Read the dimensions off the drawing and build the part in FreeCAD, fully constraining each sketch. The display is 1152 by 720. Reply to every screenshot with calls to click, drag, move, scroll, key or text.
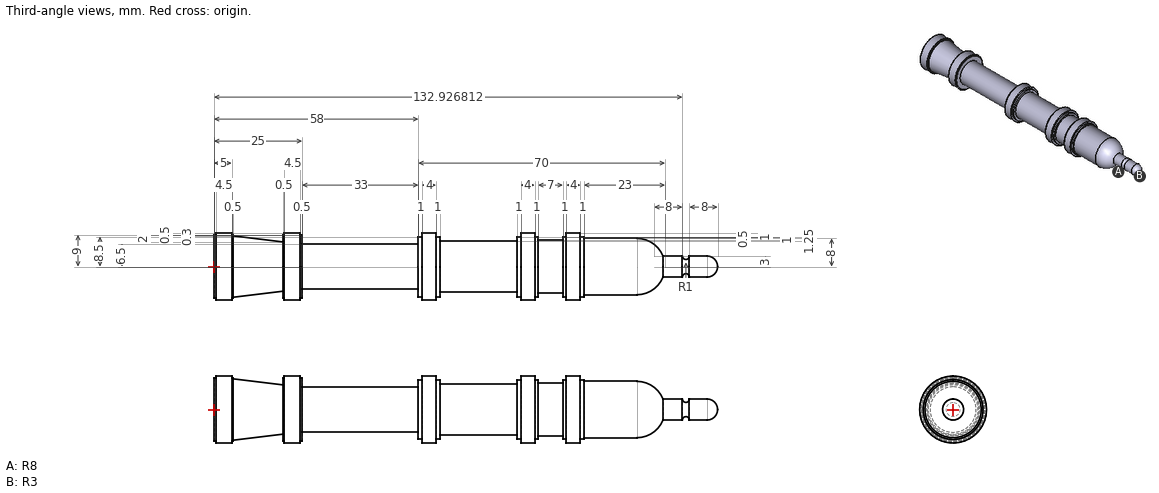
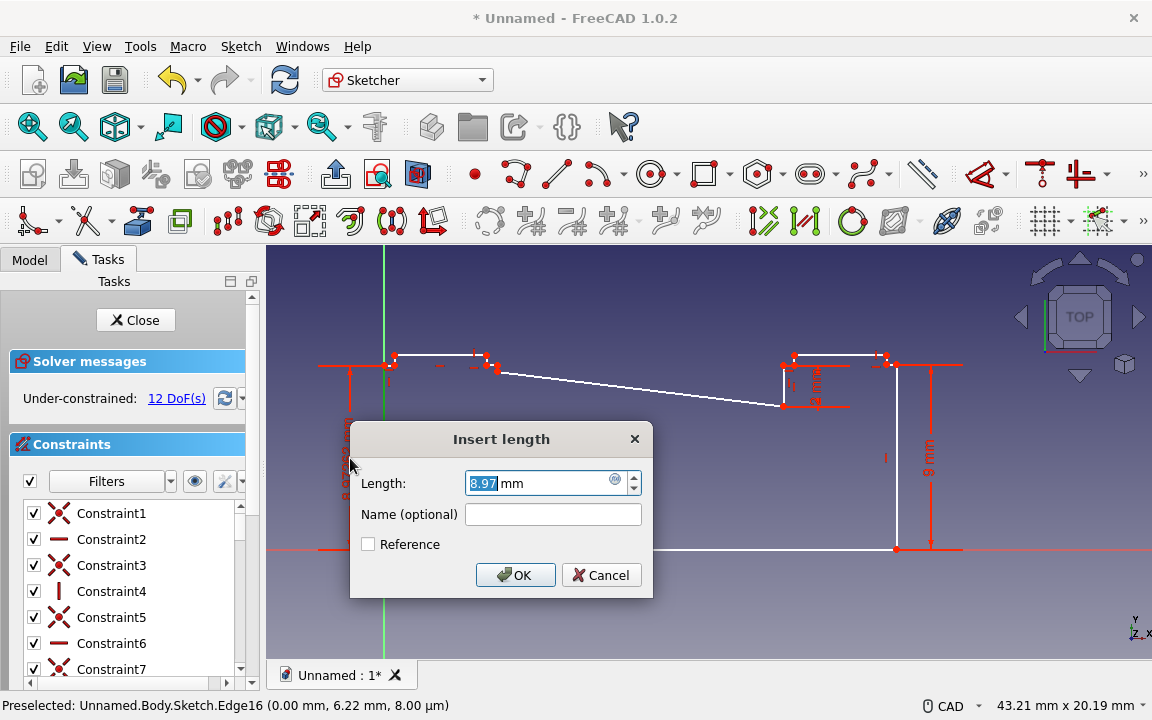
text(9)
key(Return)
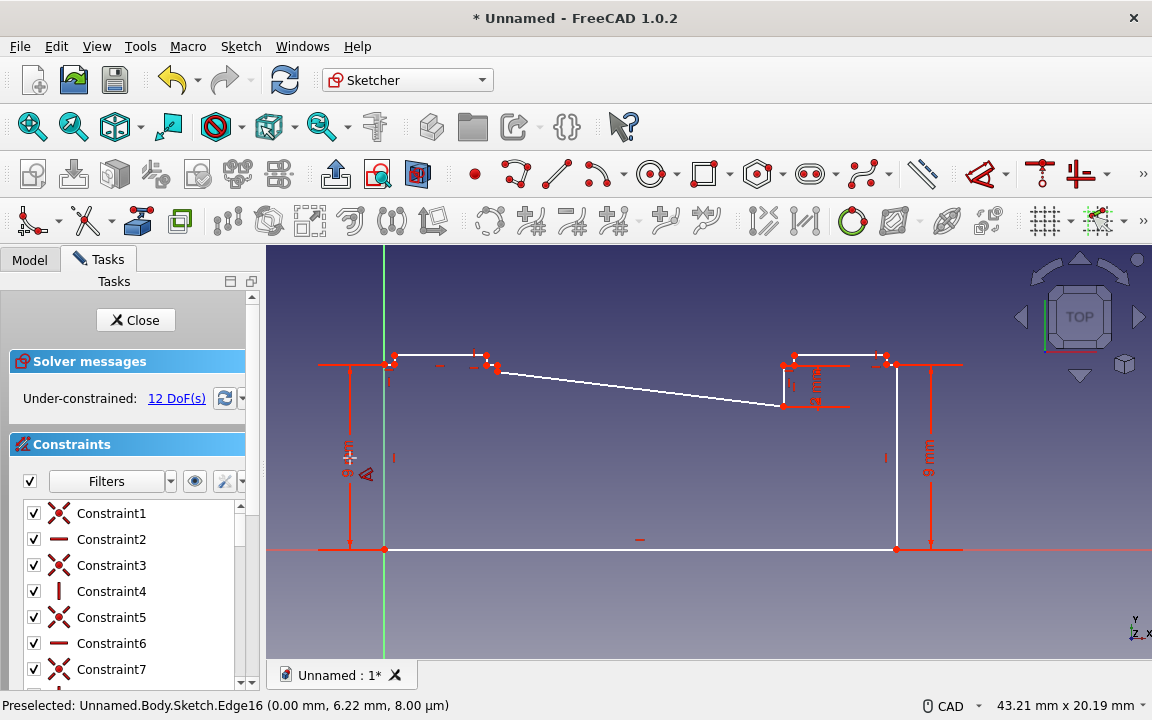
click(538, 550)
click(641, 584)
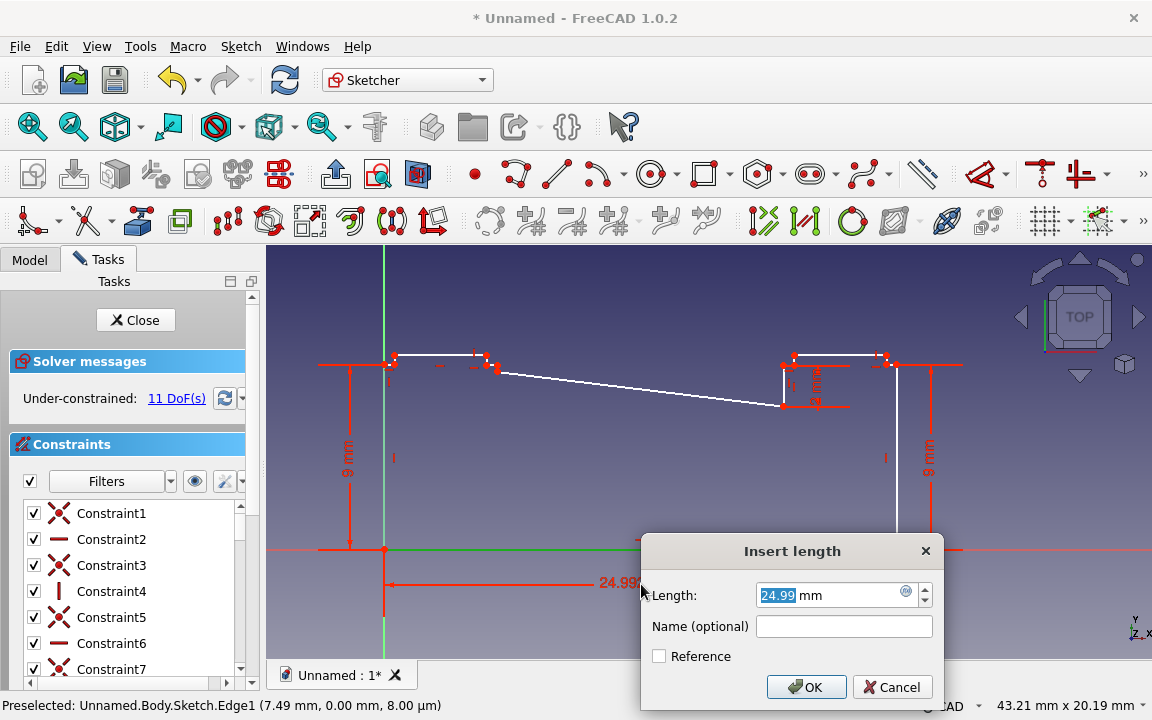
text(25)
key(Return)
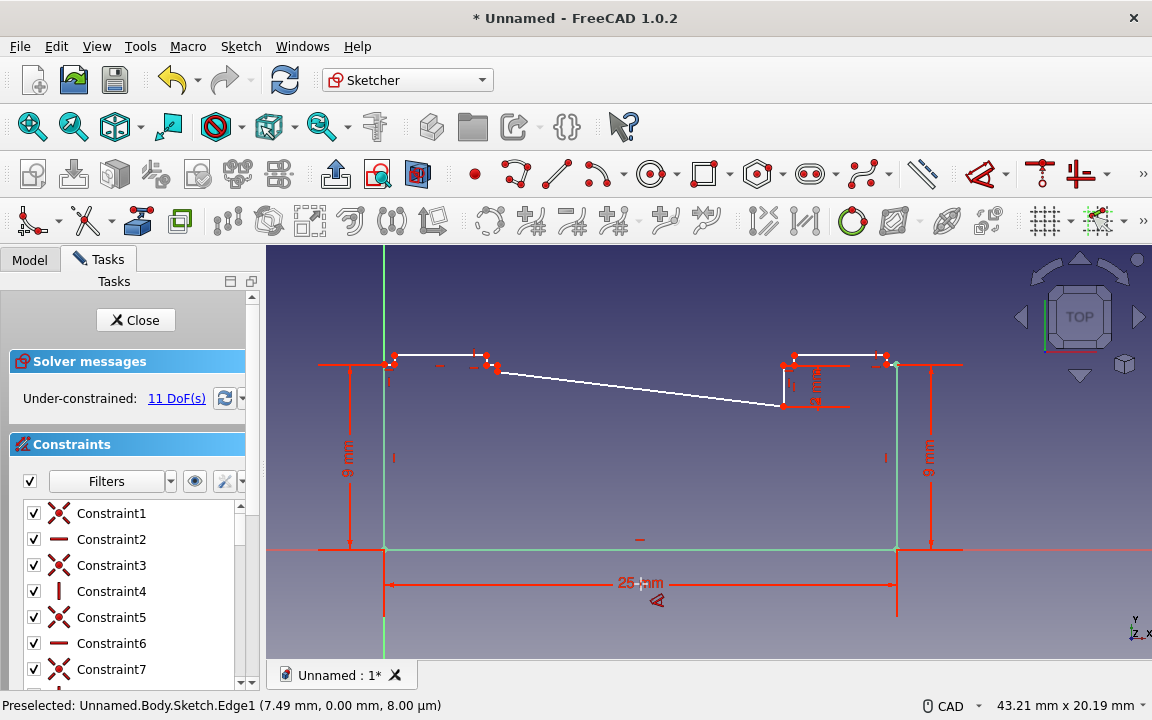
click(794, 366)
click(350, 415)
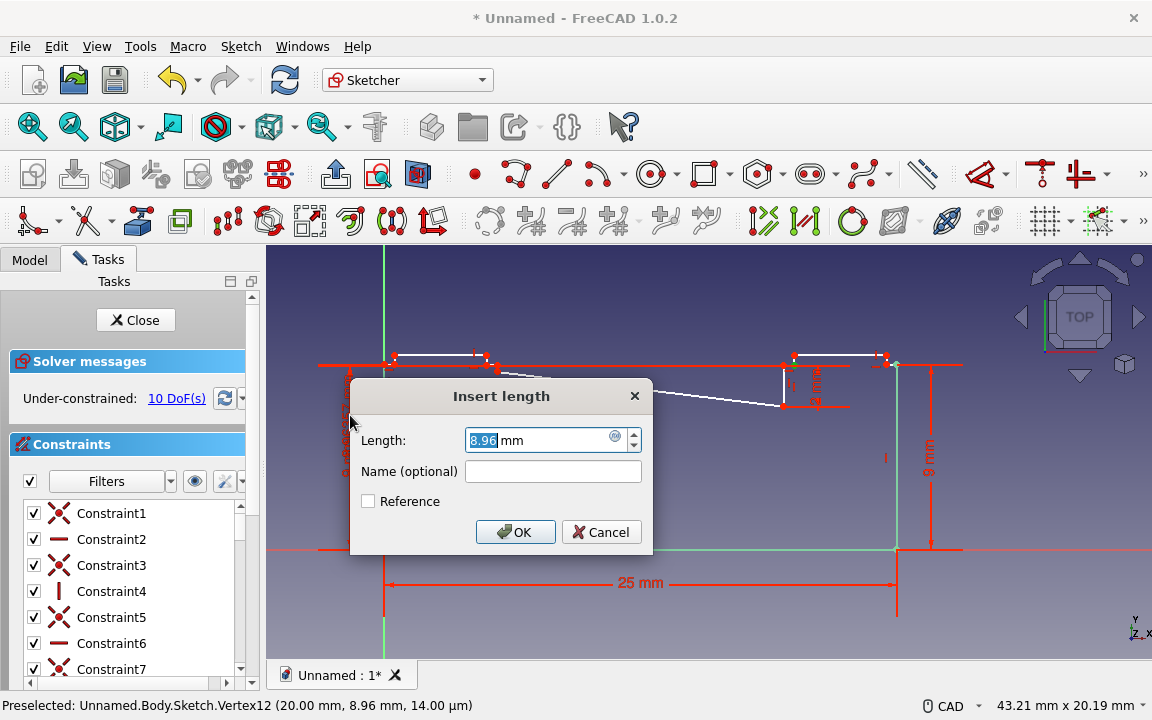
text(9)
key(Return)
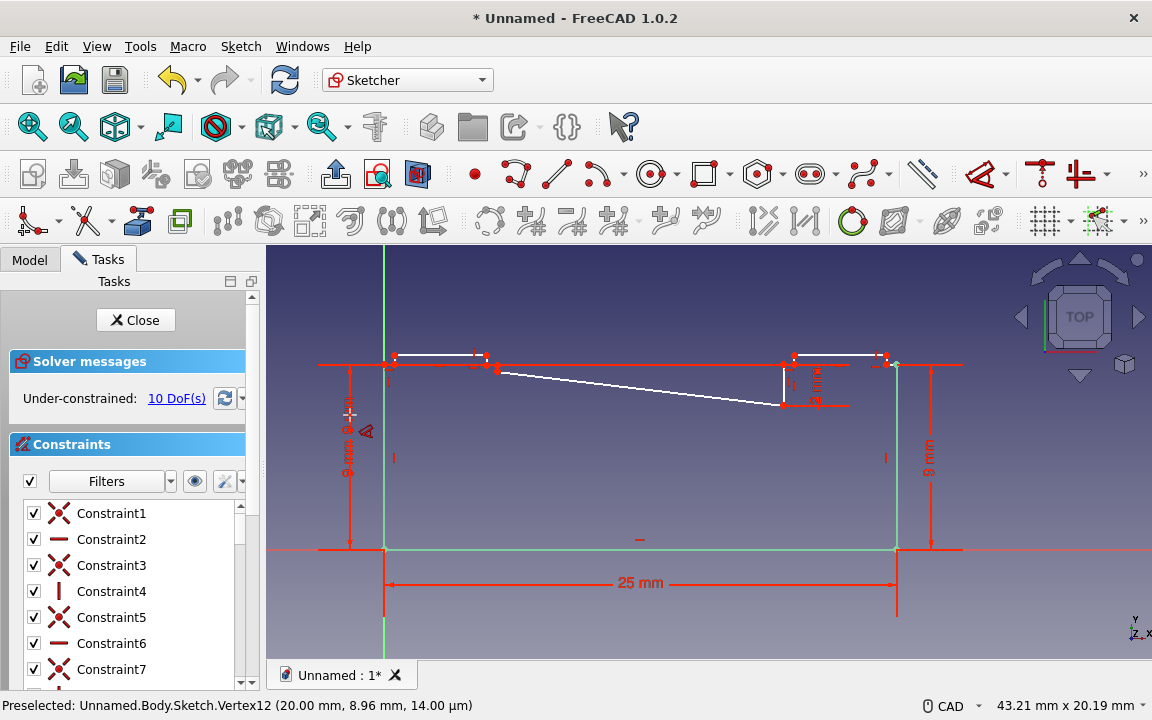
scroll(497, 365, up, 3)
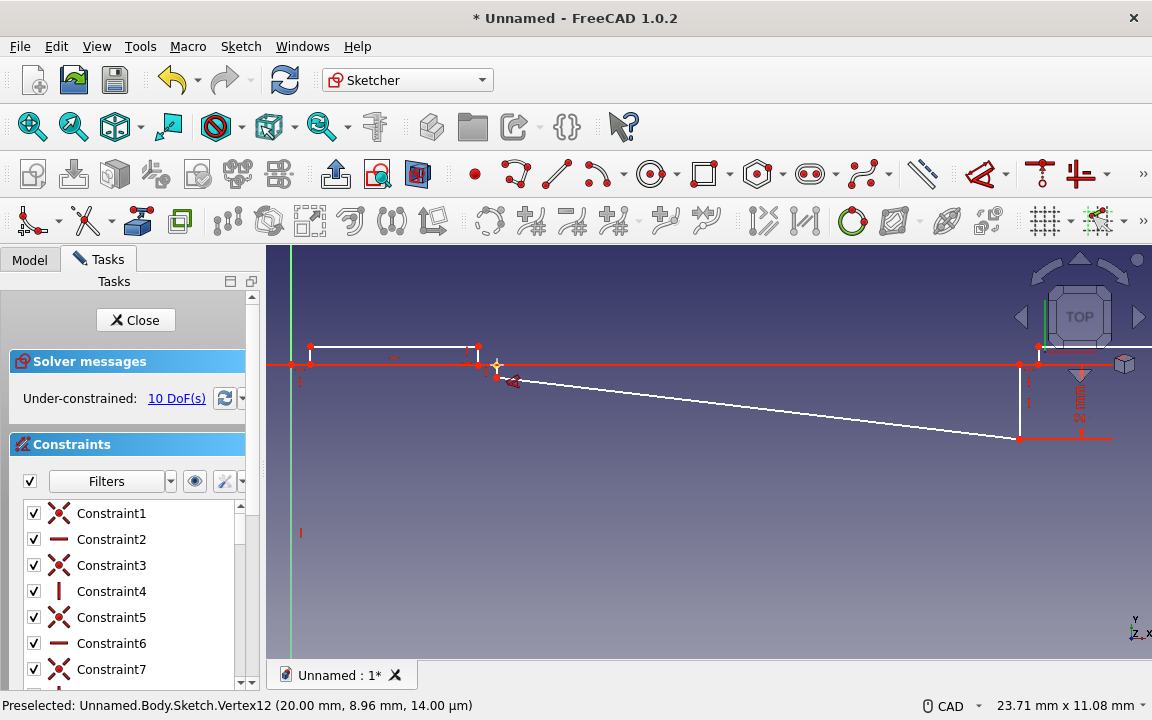
click(497, 365)
click(531, 498)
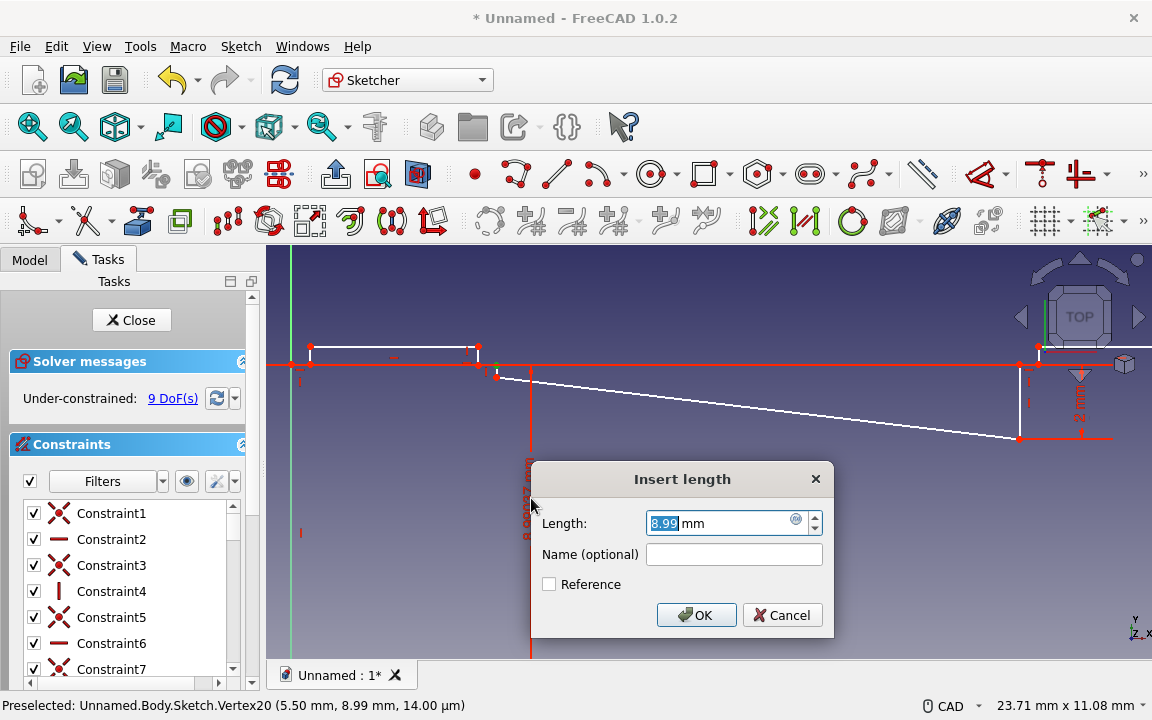
text(9)
key(Return)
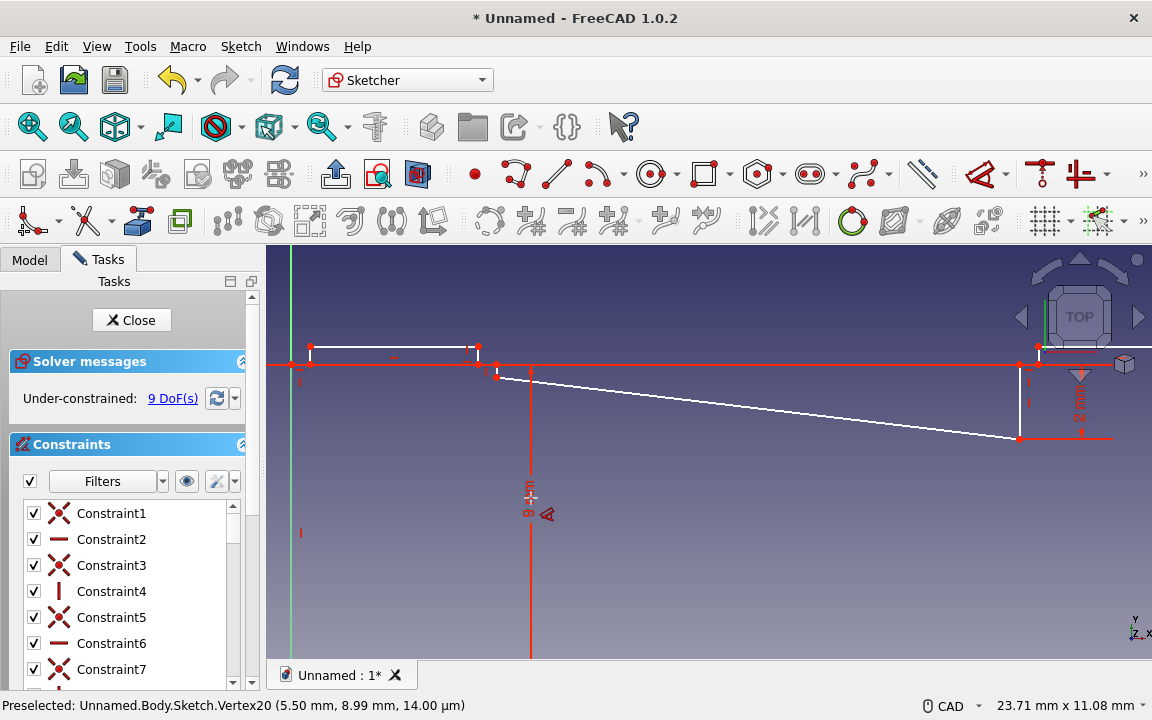
click(478, 365)
click(386, 331)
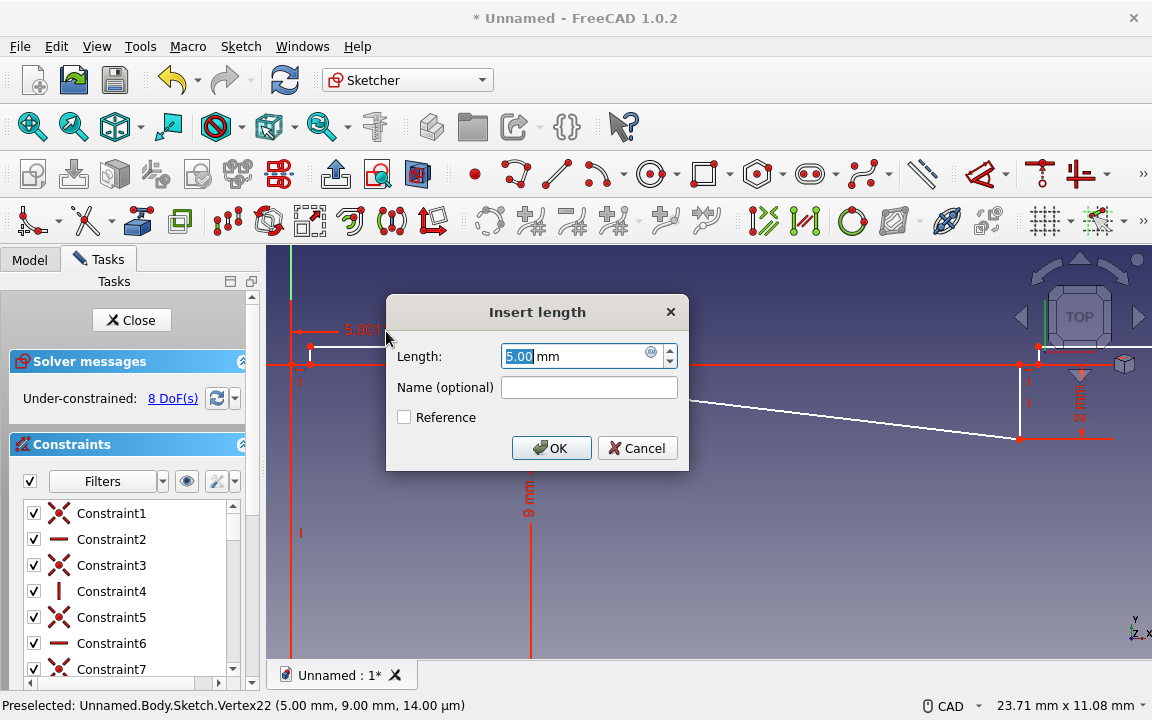
text(5)
key(Return)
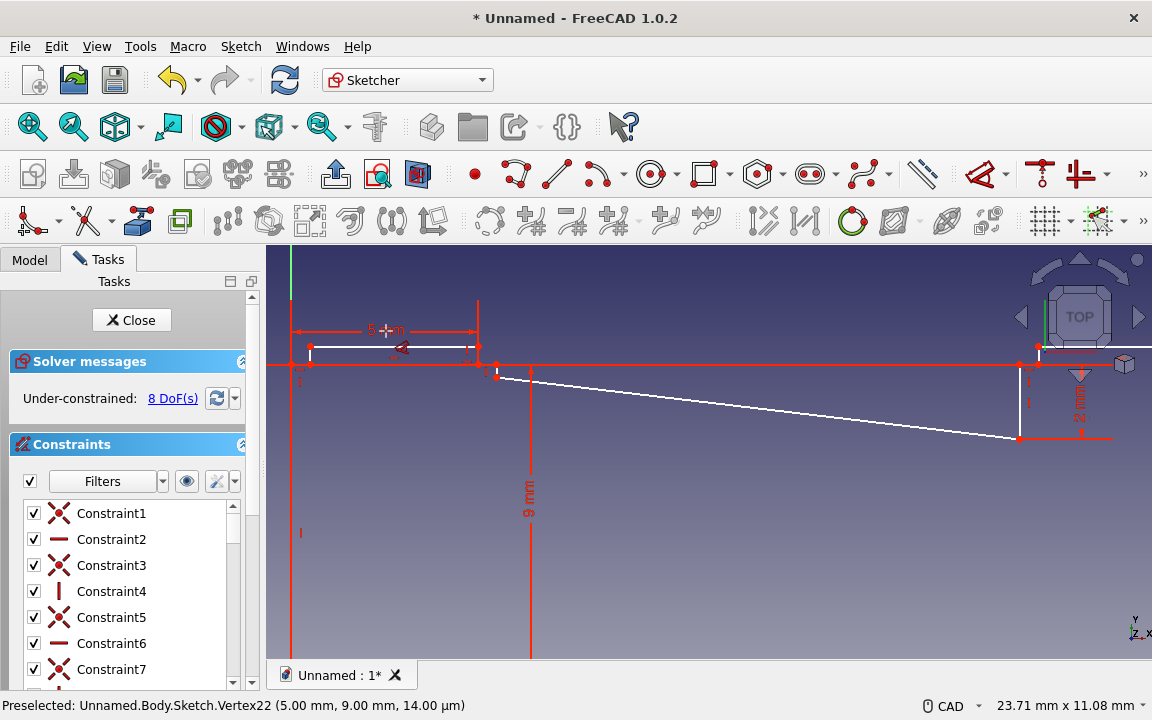
scroll(497, 365, down, 3)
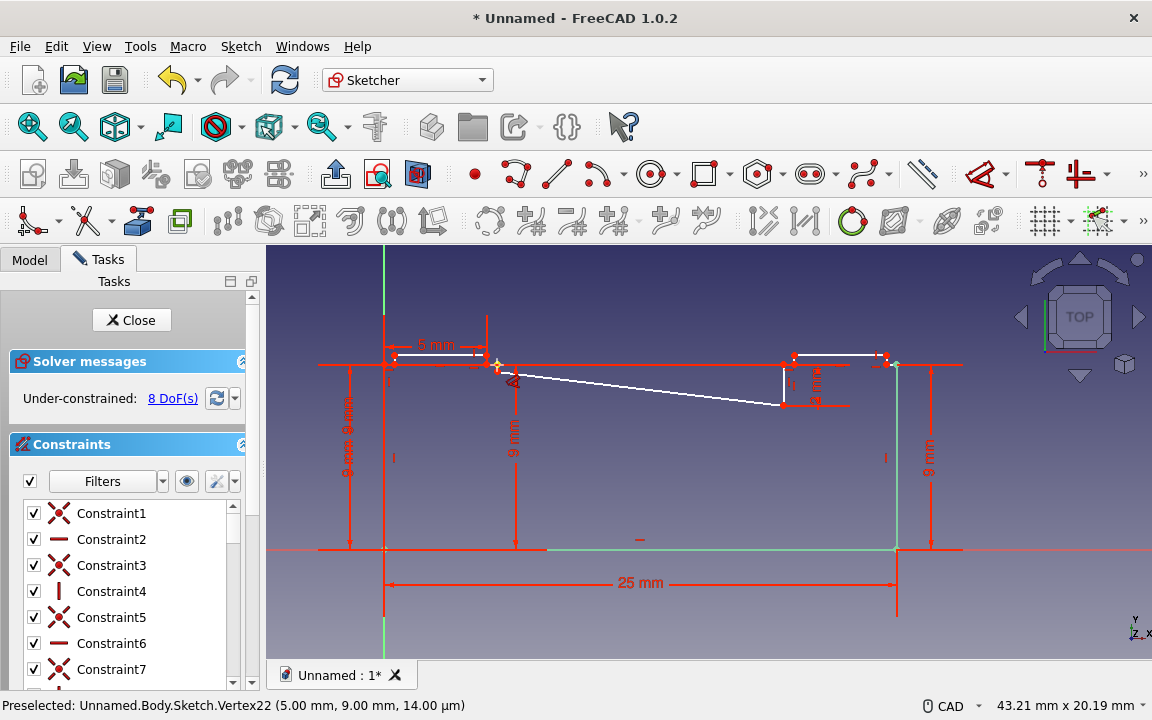
scroll(892, 365, up, 7)